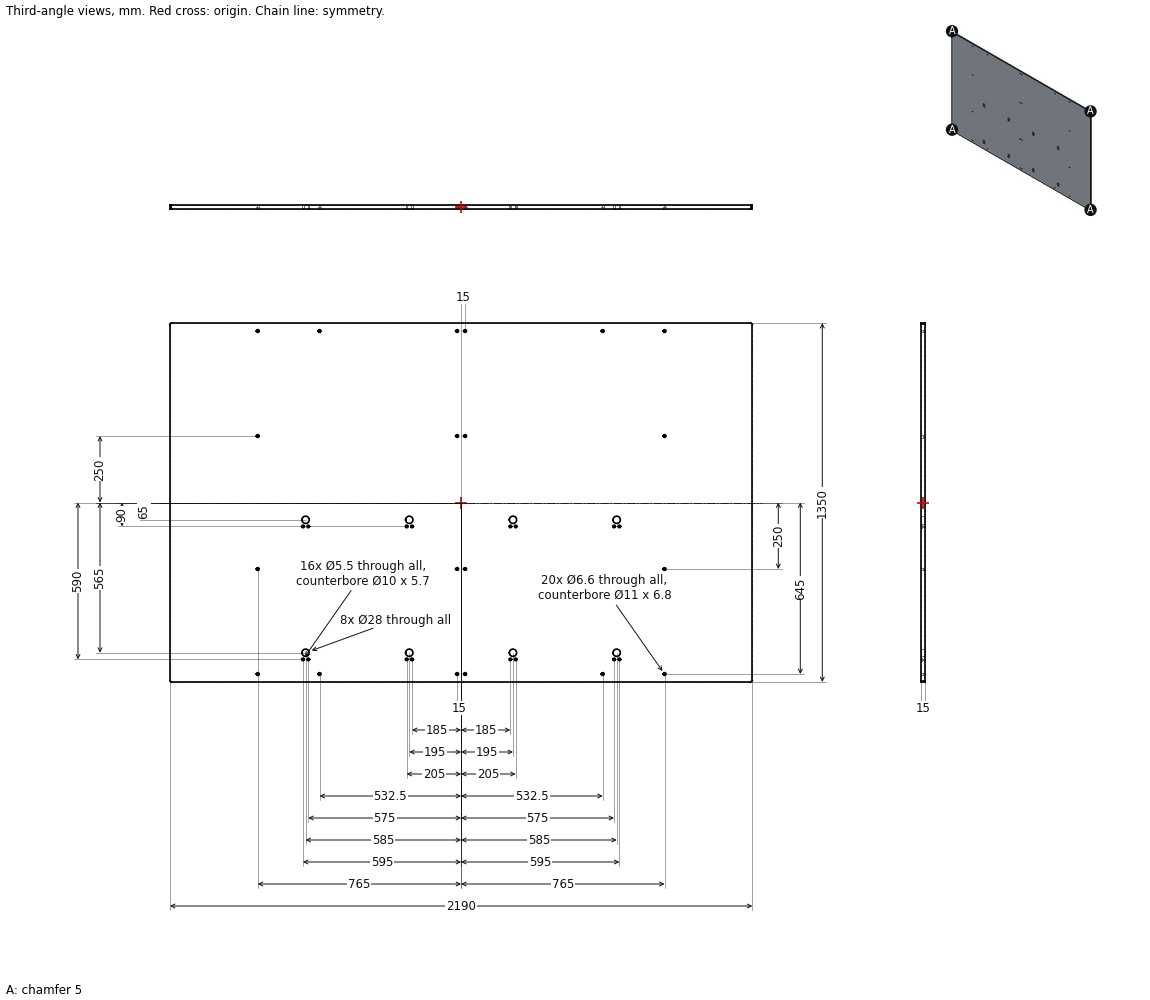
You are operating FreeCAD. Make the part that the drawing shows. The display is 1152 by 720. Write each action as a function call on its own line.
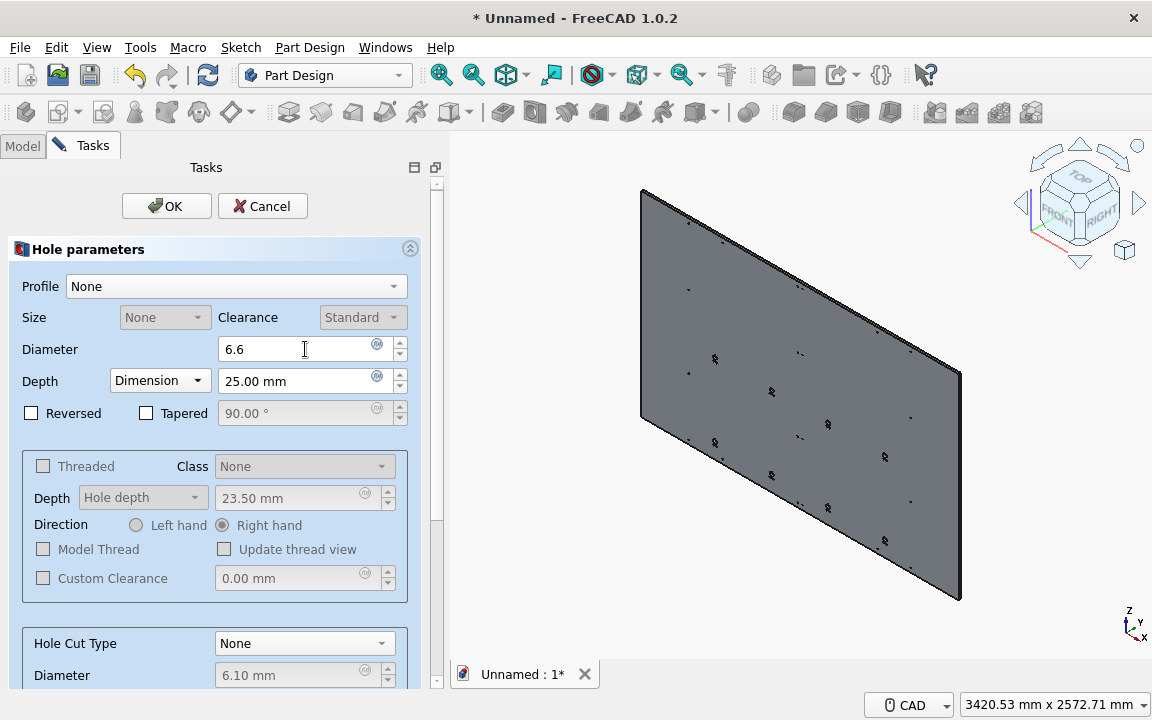
click(161, 380)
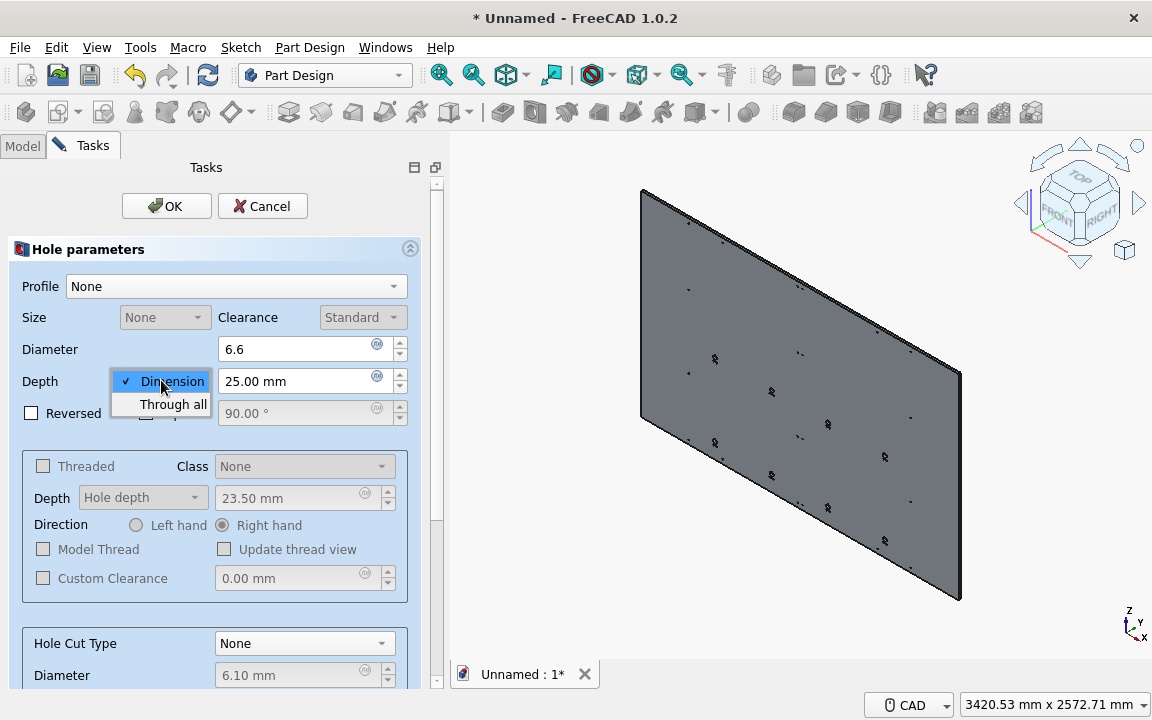
click(160, 404)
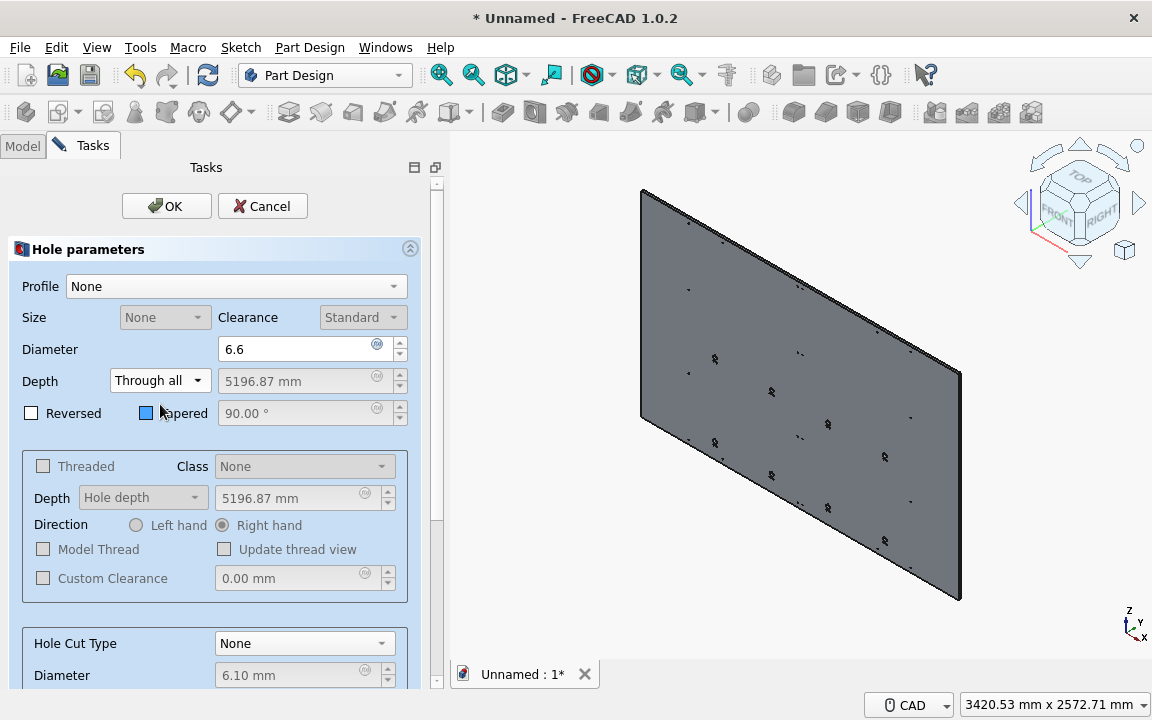
click(306, 644)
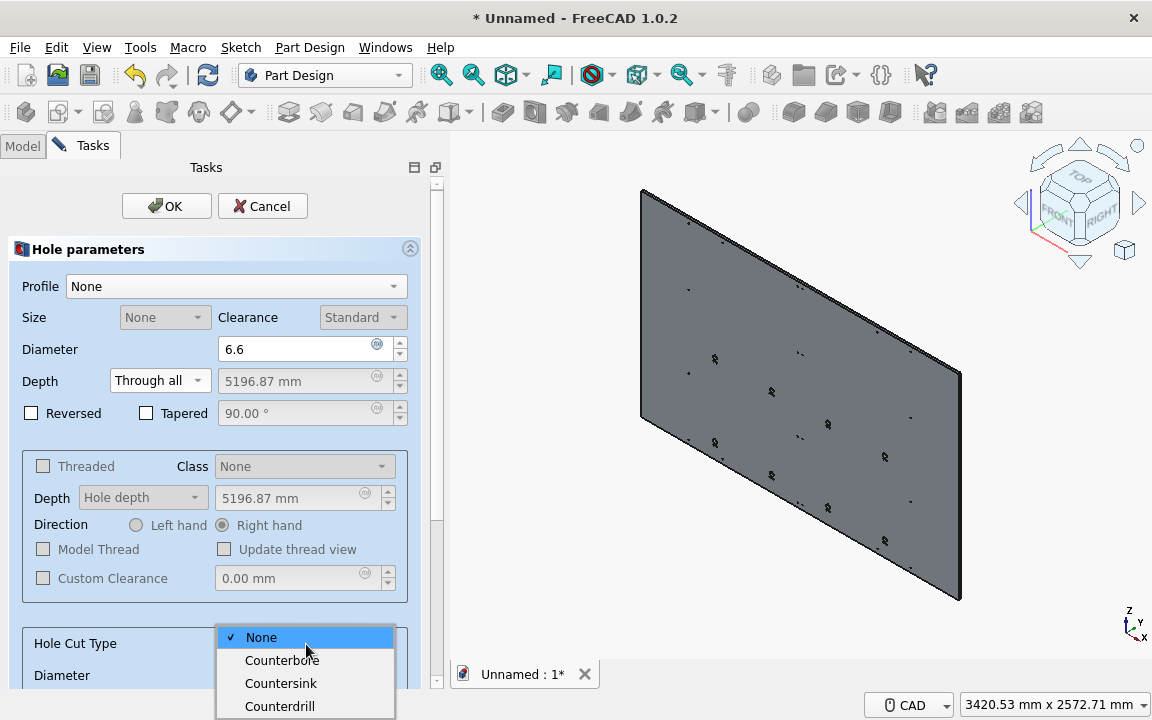
click(304, 660)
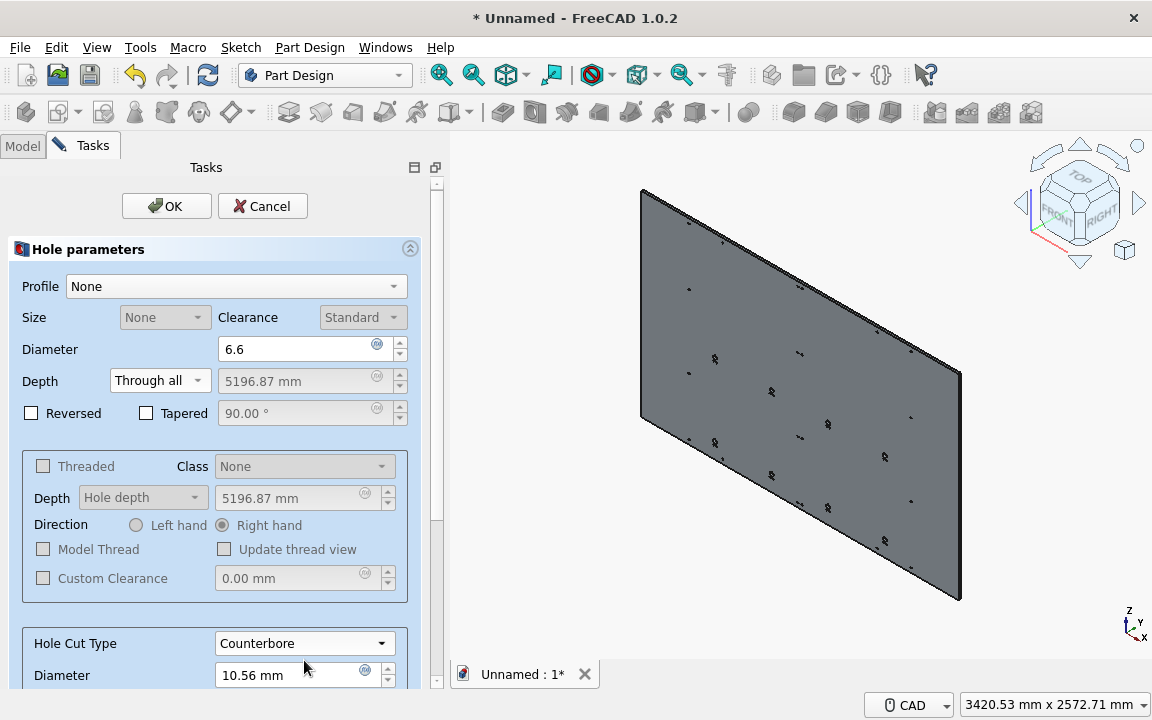
triple_click(298, 675)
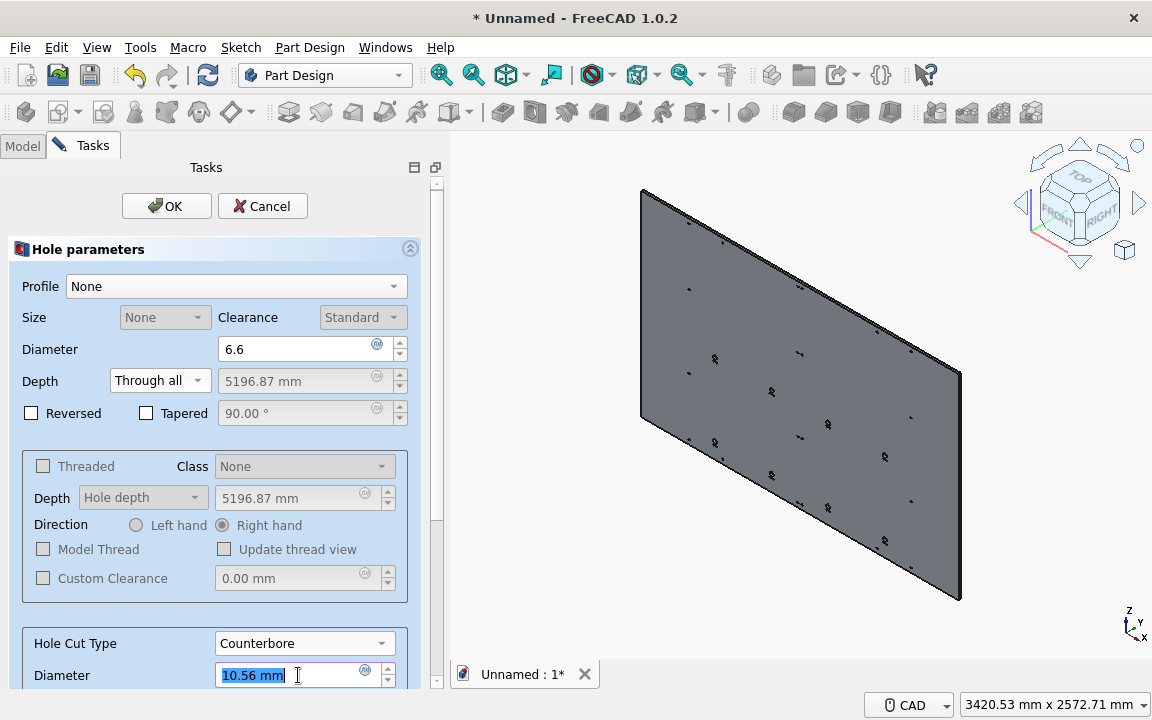
text(11)
key(Tab)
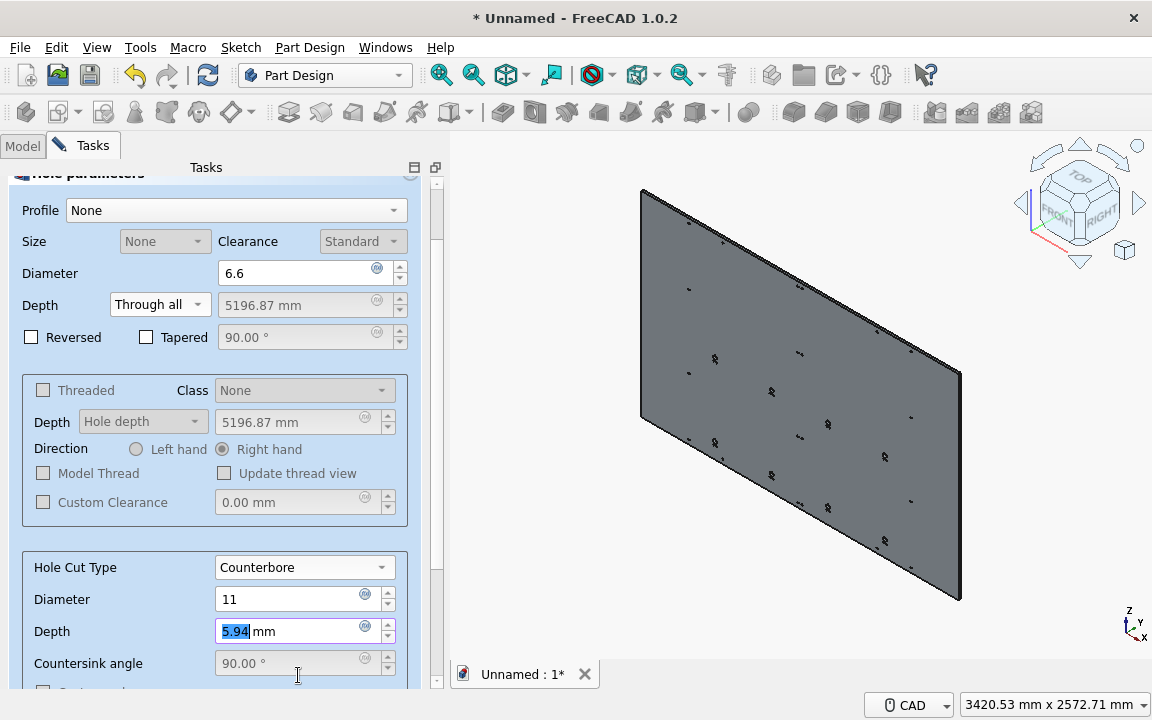
text(6.8)
key(Tab)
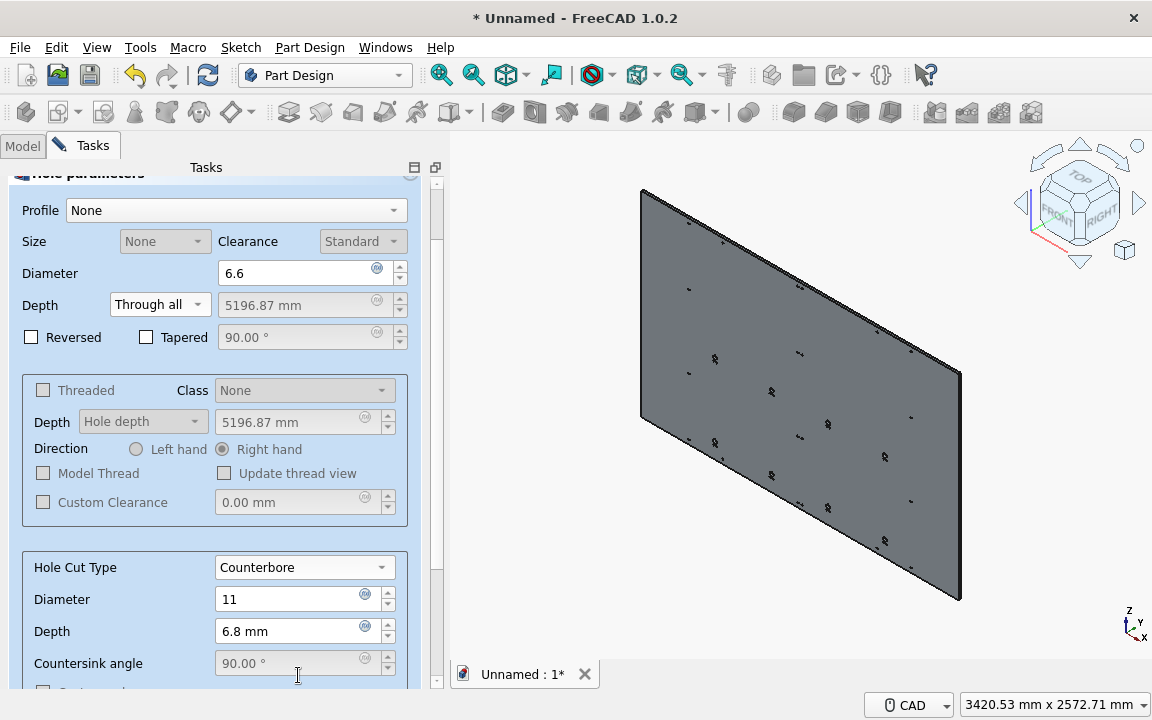
scroll(437, 432, up, 3)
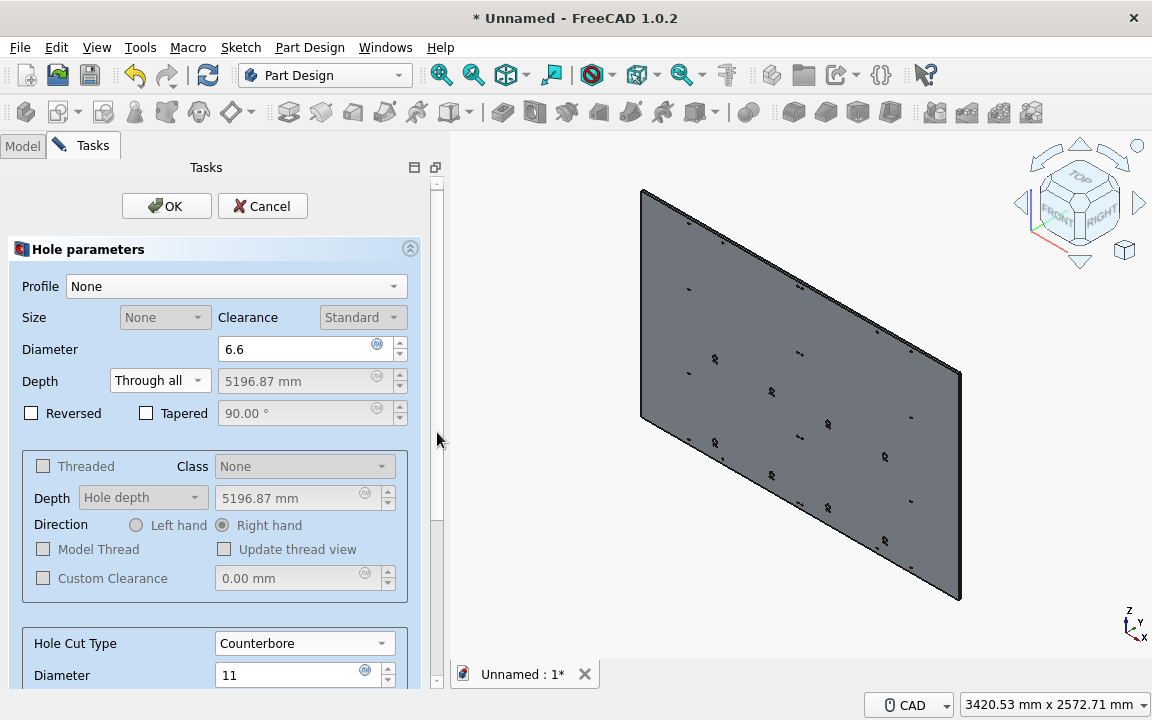
click(167, 206)